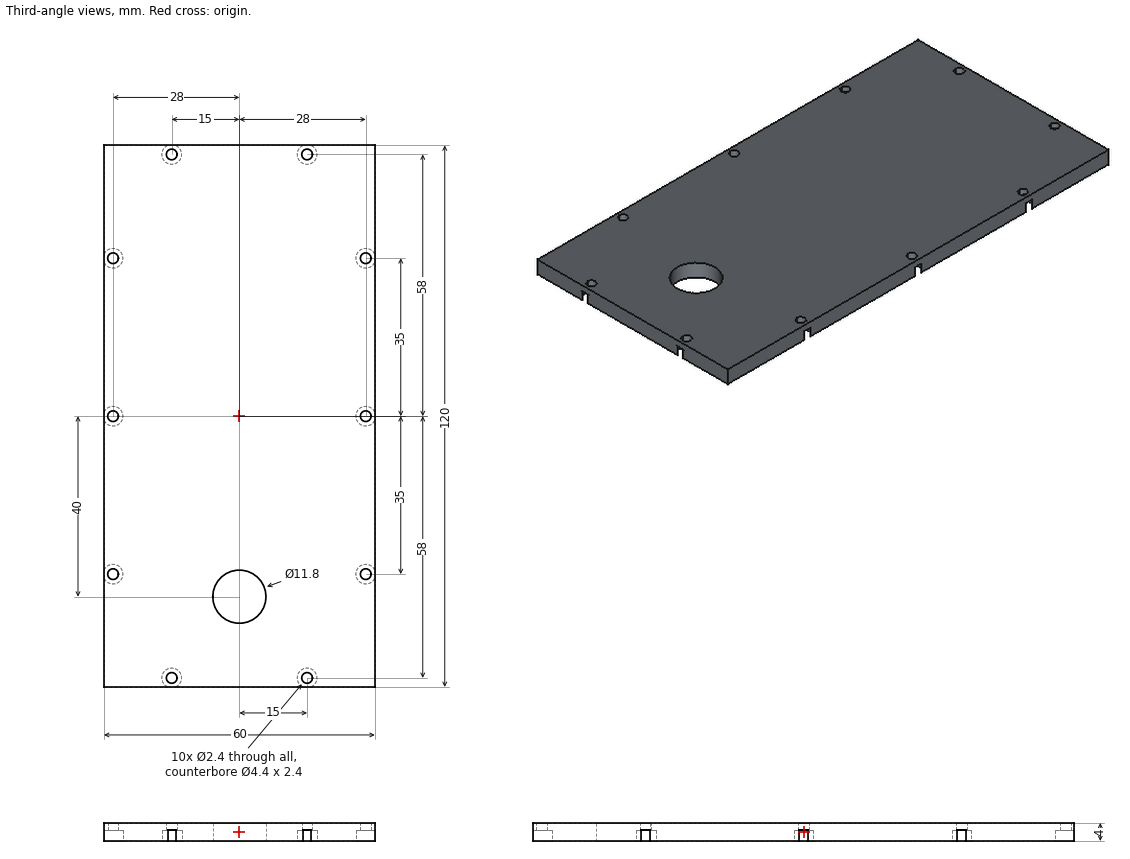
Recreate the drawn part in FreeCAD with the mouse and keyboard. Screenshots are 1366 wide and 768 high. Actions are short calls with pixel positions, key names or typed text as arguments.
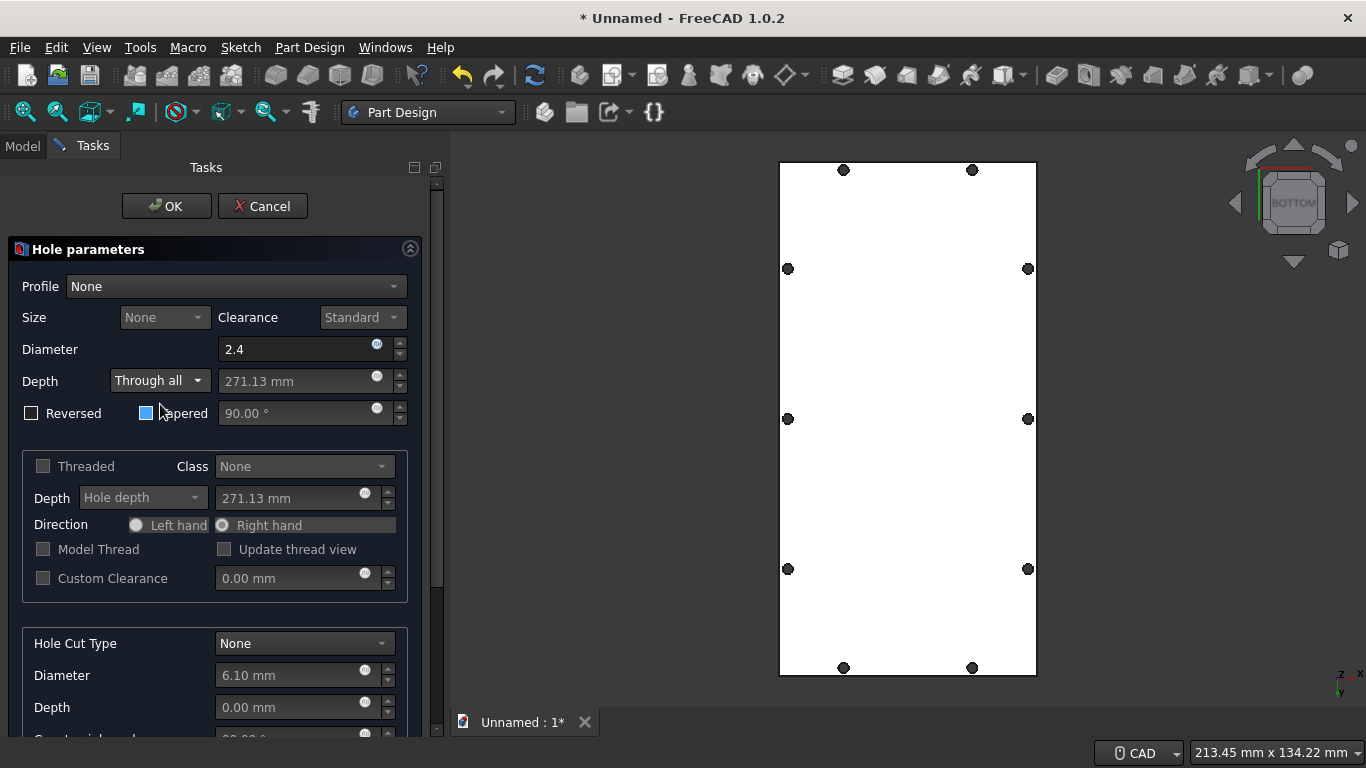
click(306, 644)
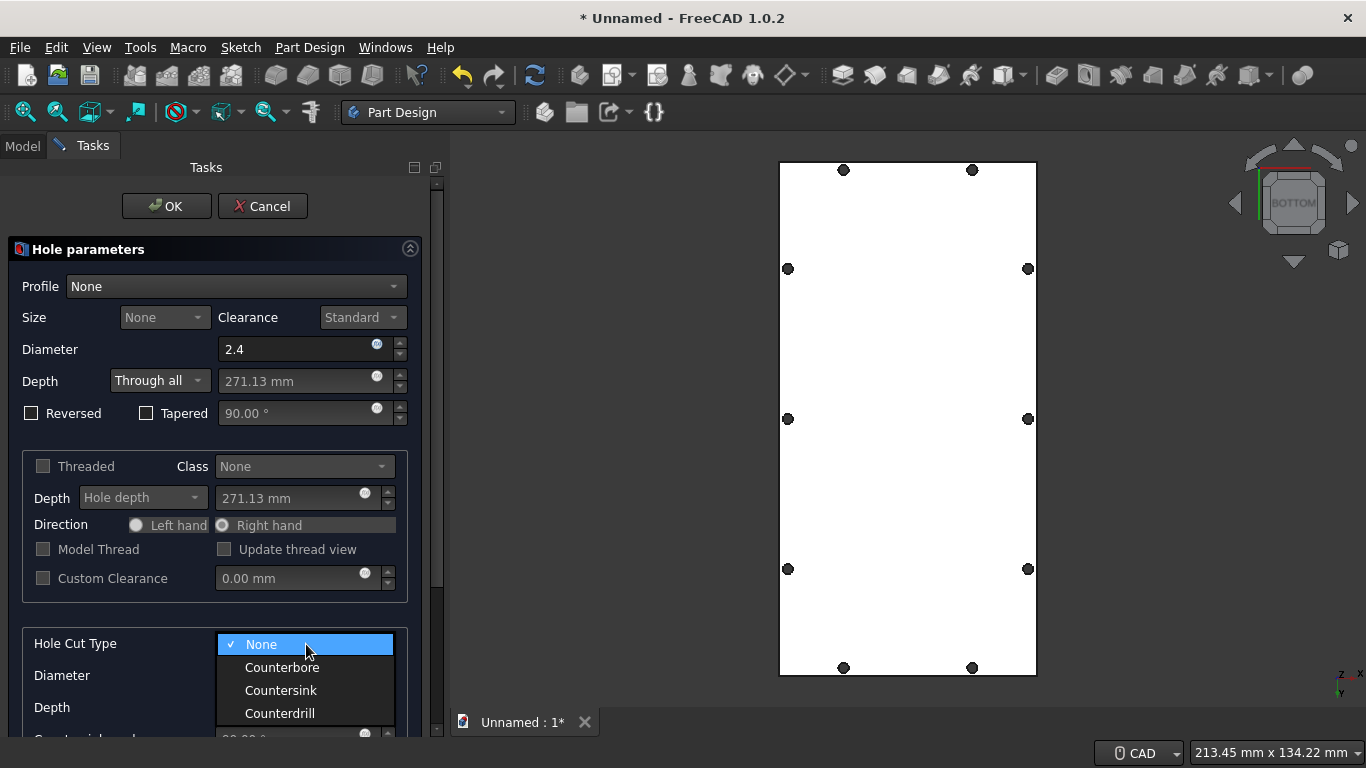
click(304, 668)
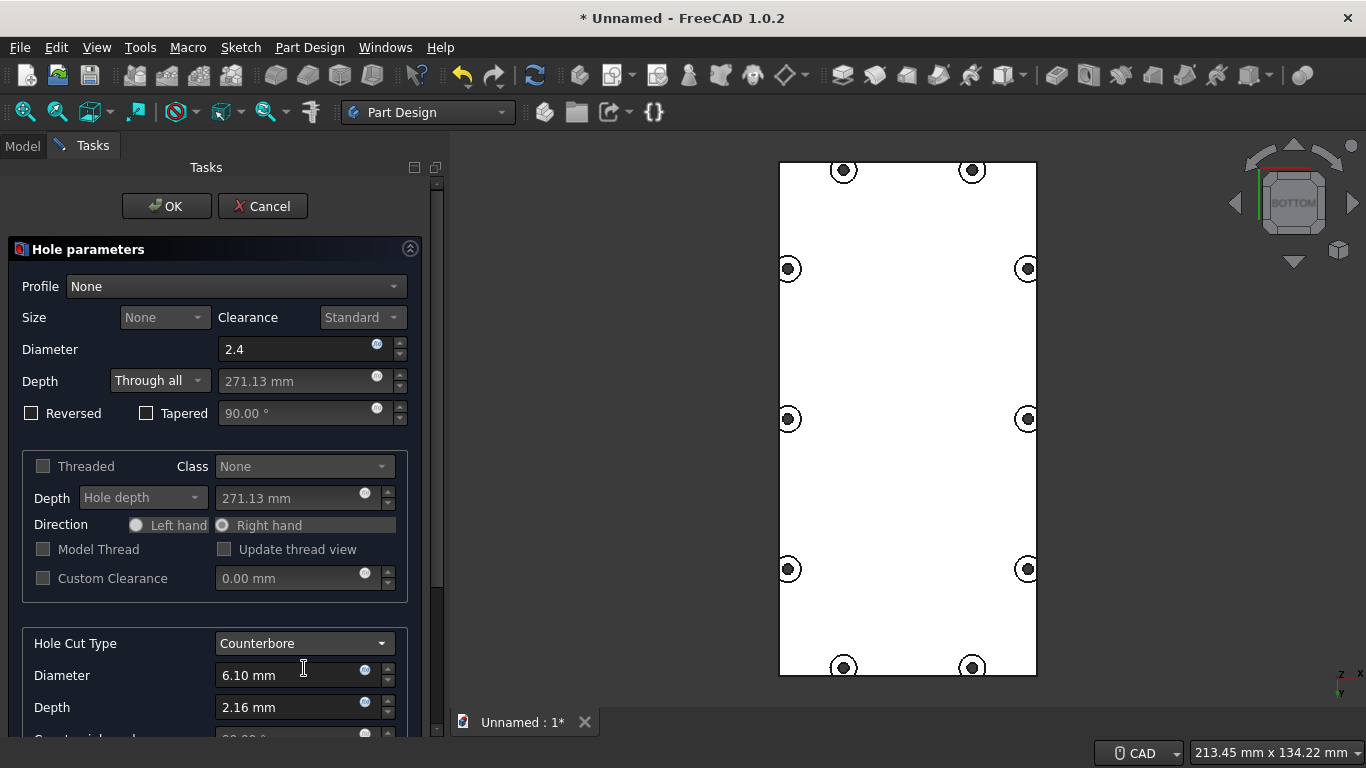
triple_click(298, 675)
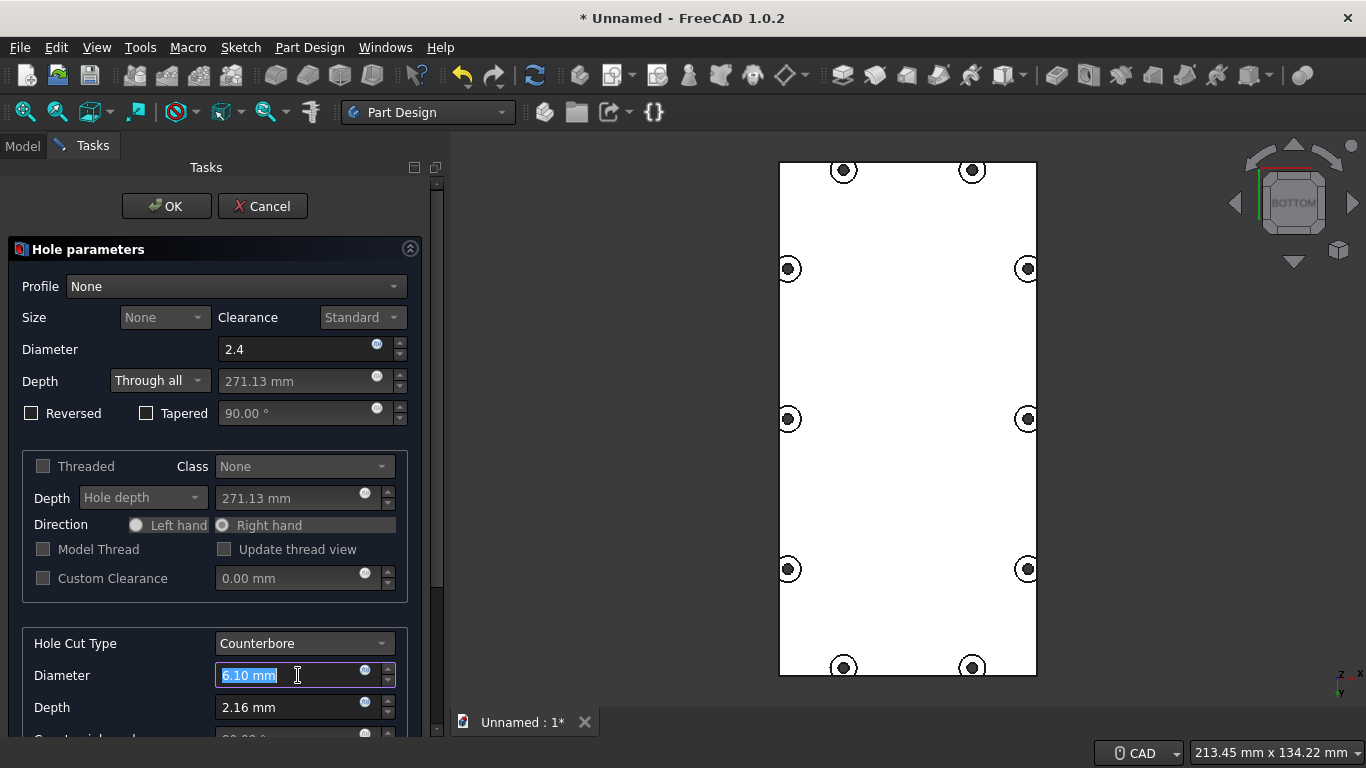
text(4.4)
key(Tab)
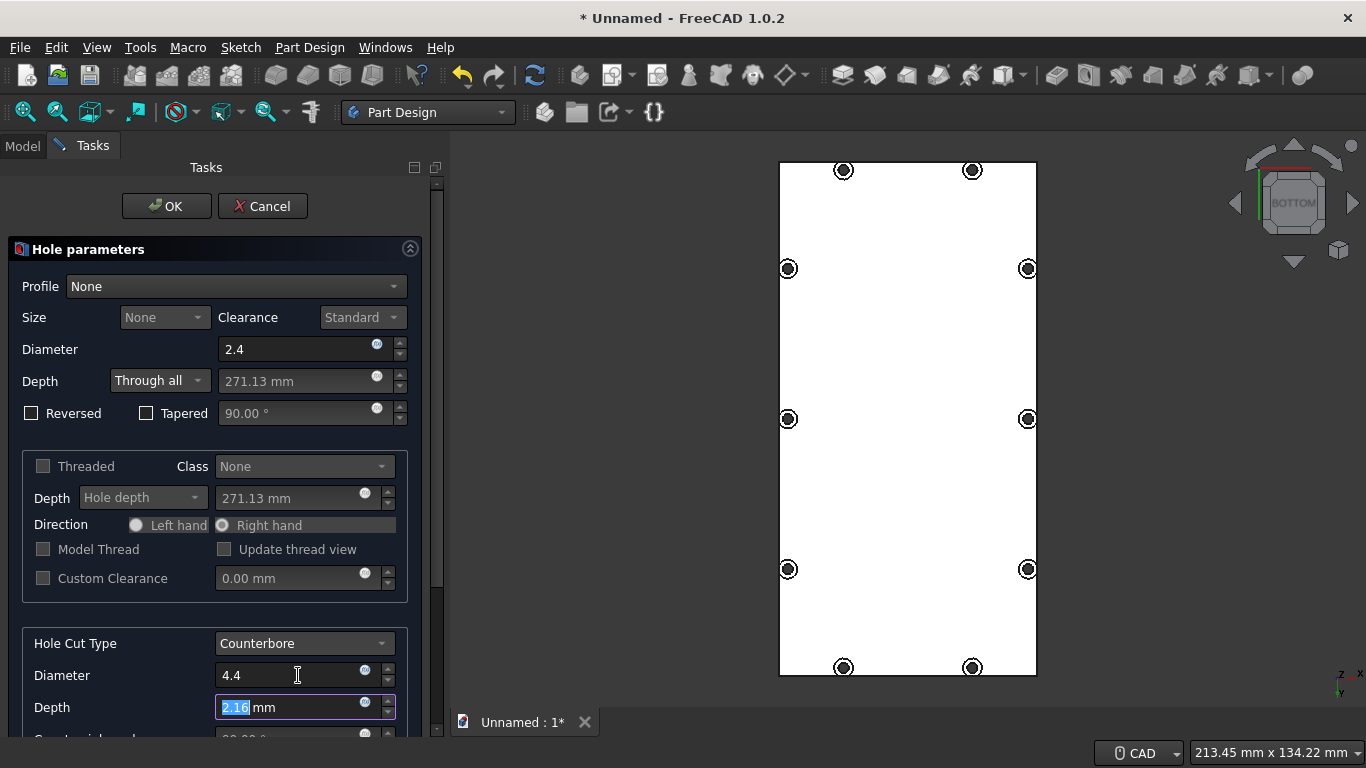
text(2.4)
key(Tab)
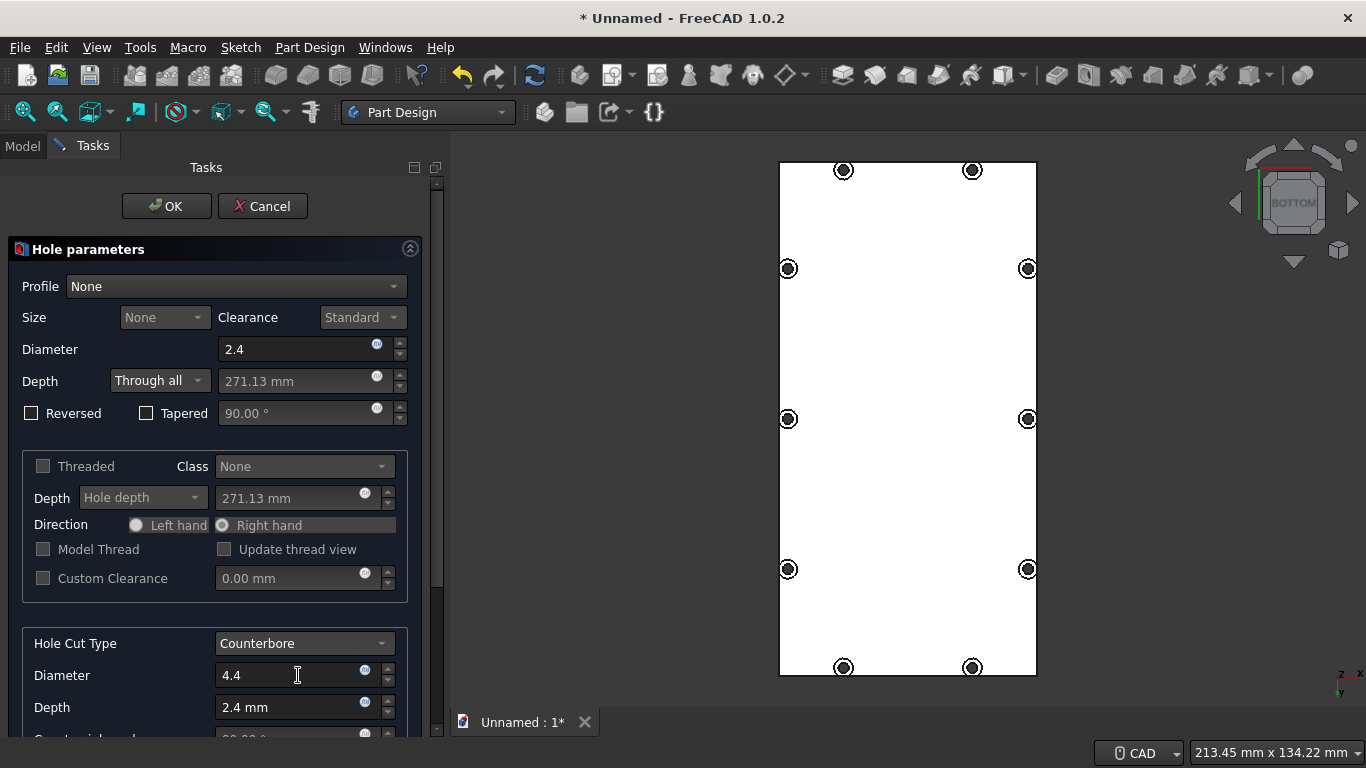
click(167, 206)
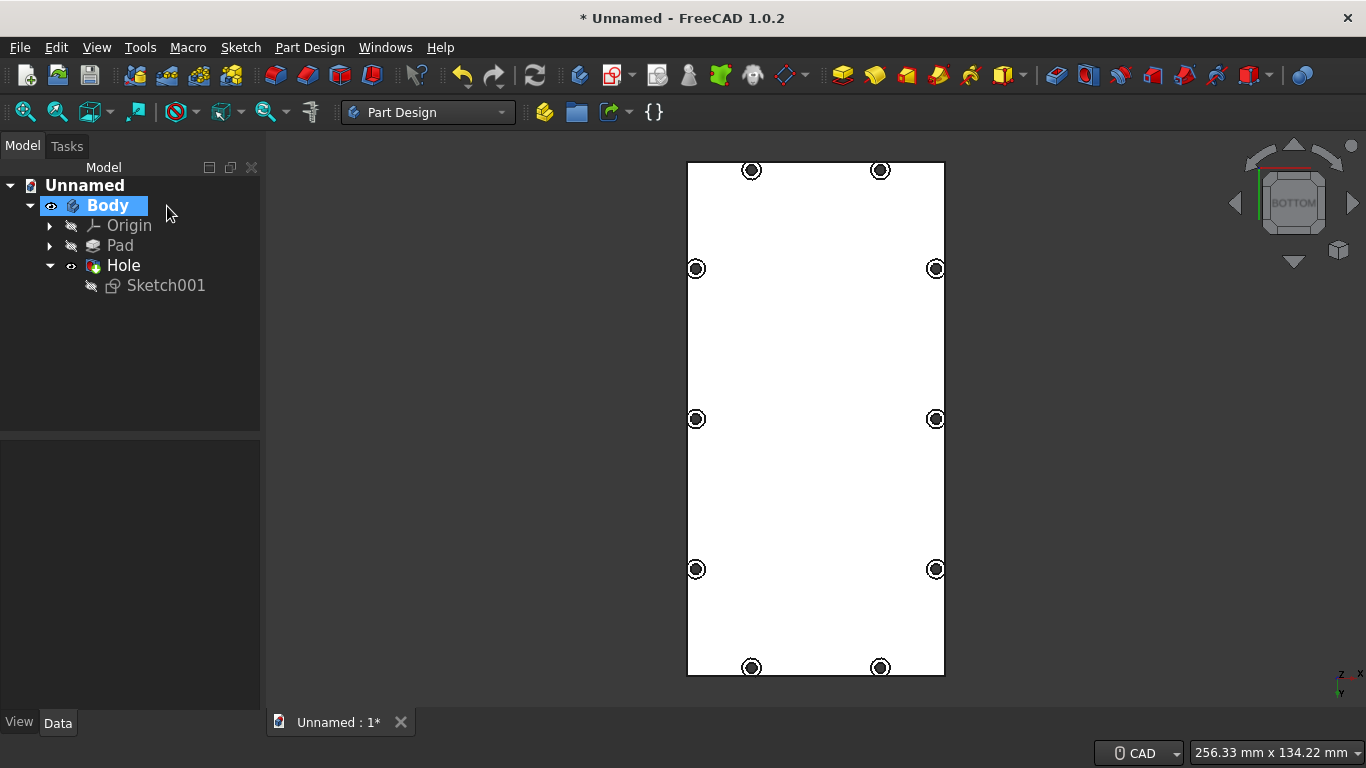
click(816, 492)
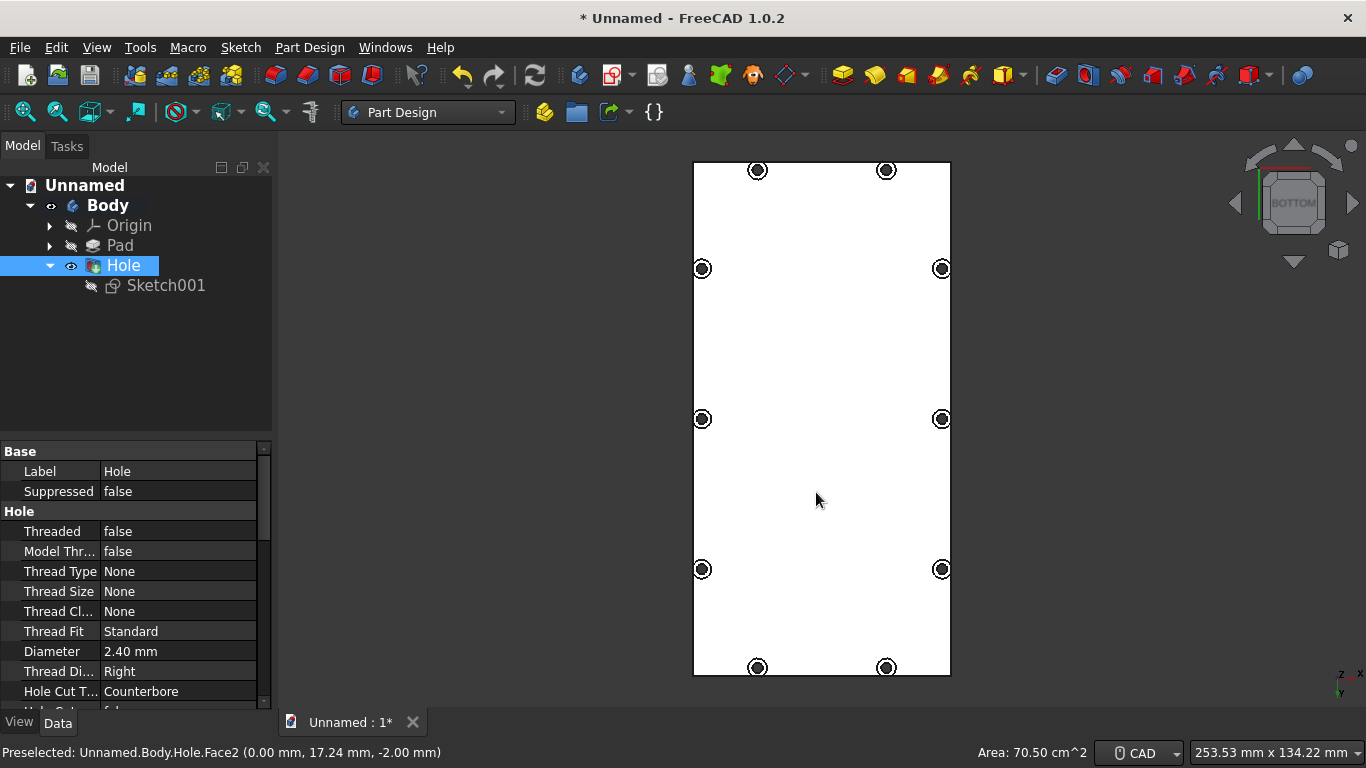
click(612, 76)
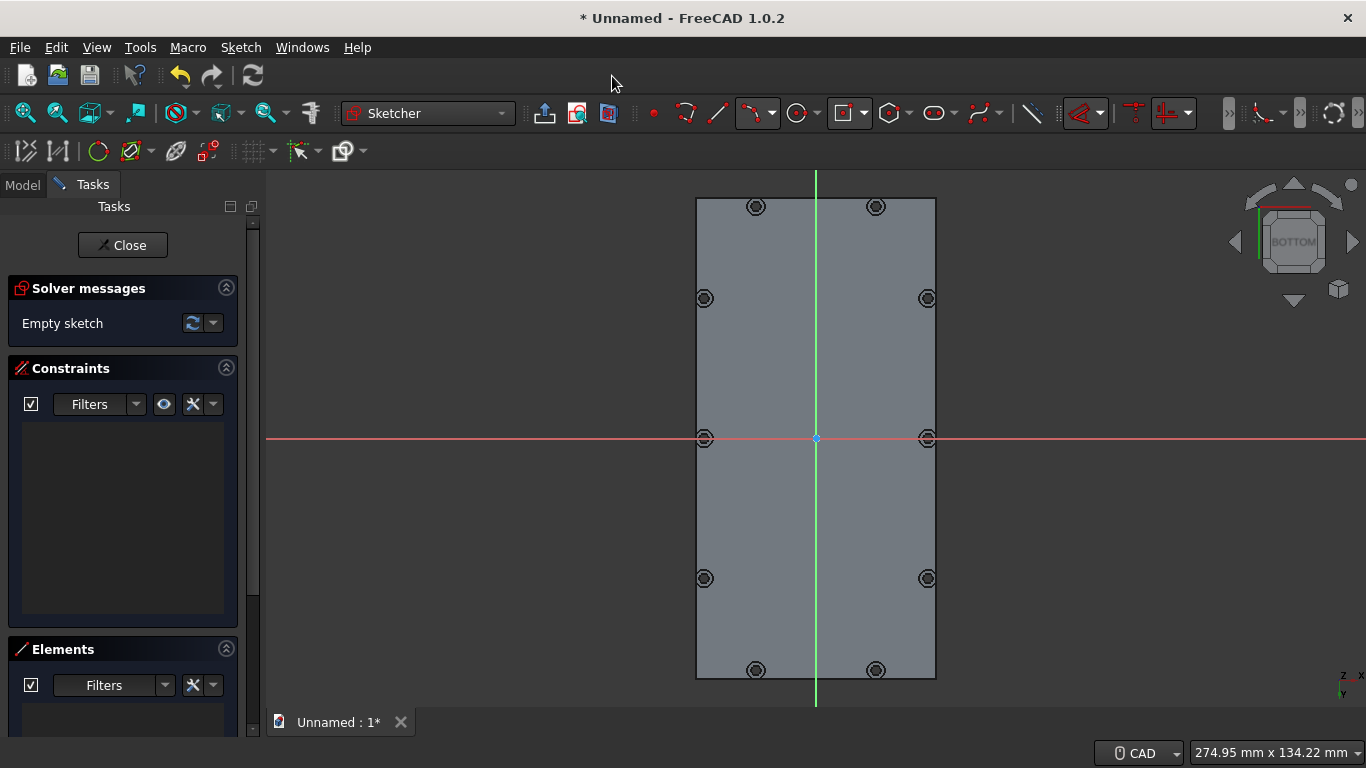
scroll(827, 253, up, 10)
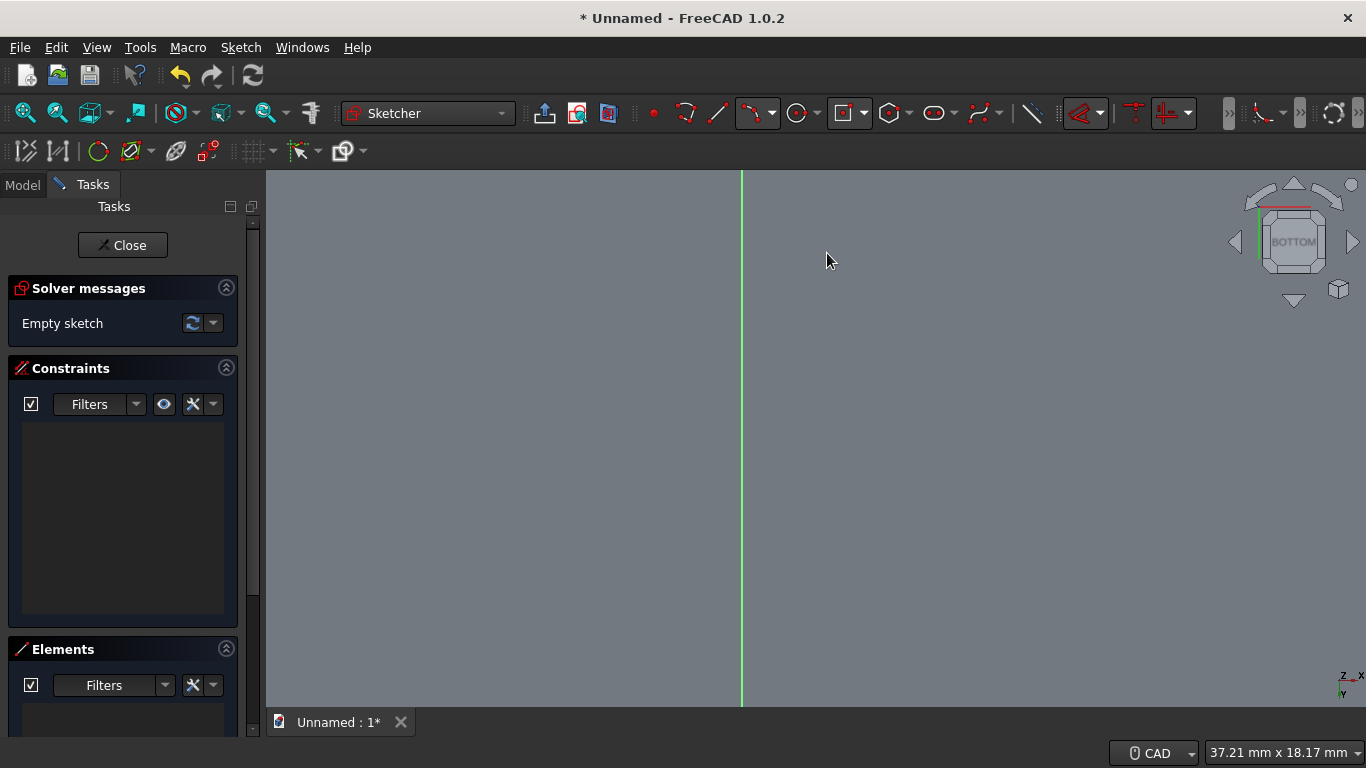
click(798, 114)